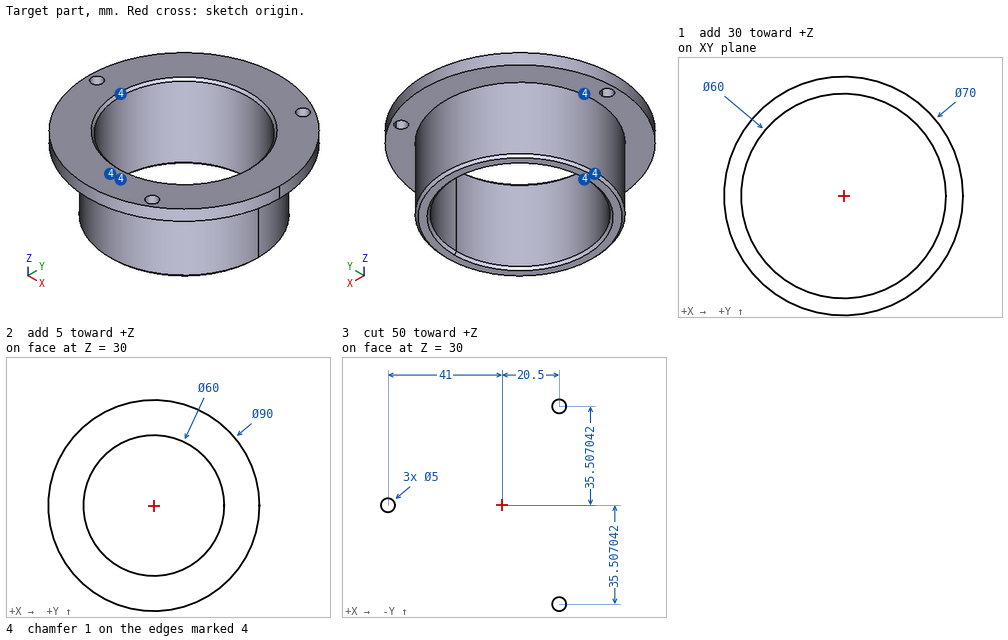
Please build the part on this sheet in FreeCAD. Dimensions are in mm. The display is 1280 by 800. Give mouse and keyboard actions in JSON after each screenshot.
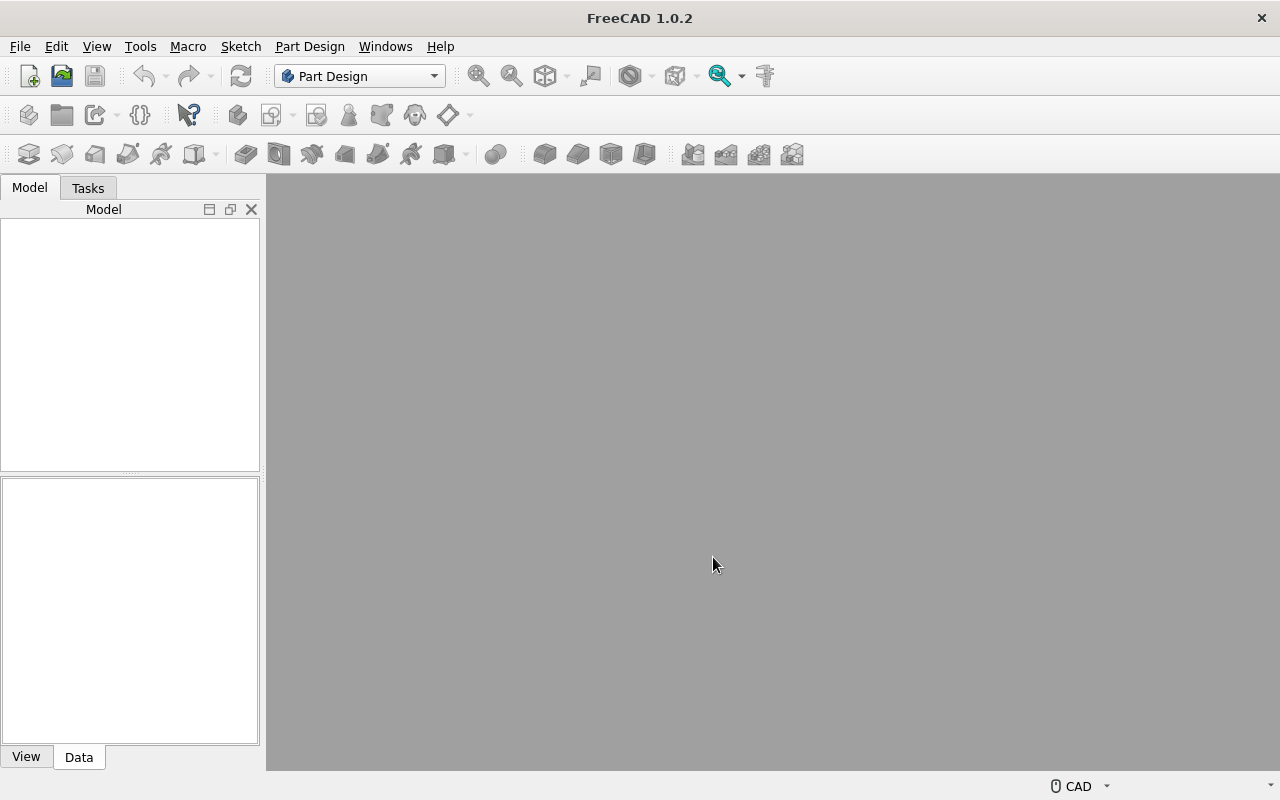
{"action": "key", "text": "ctrl+n"}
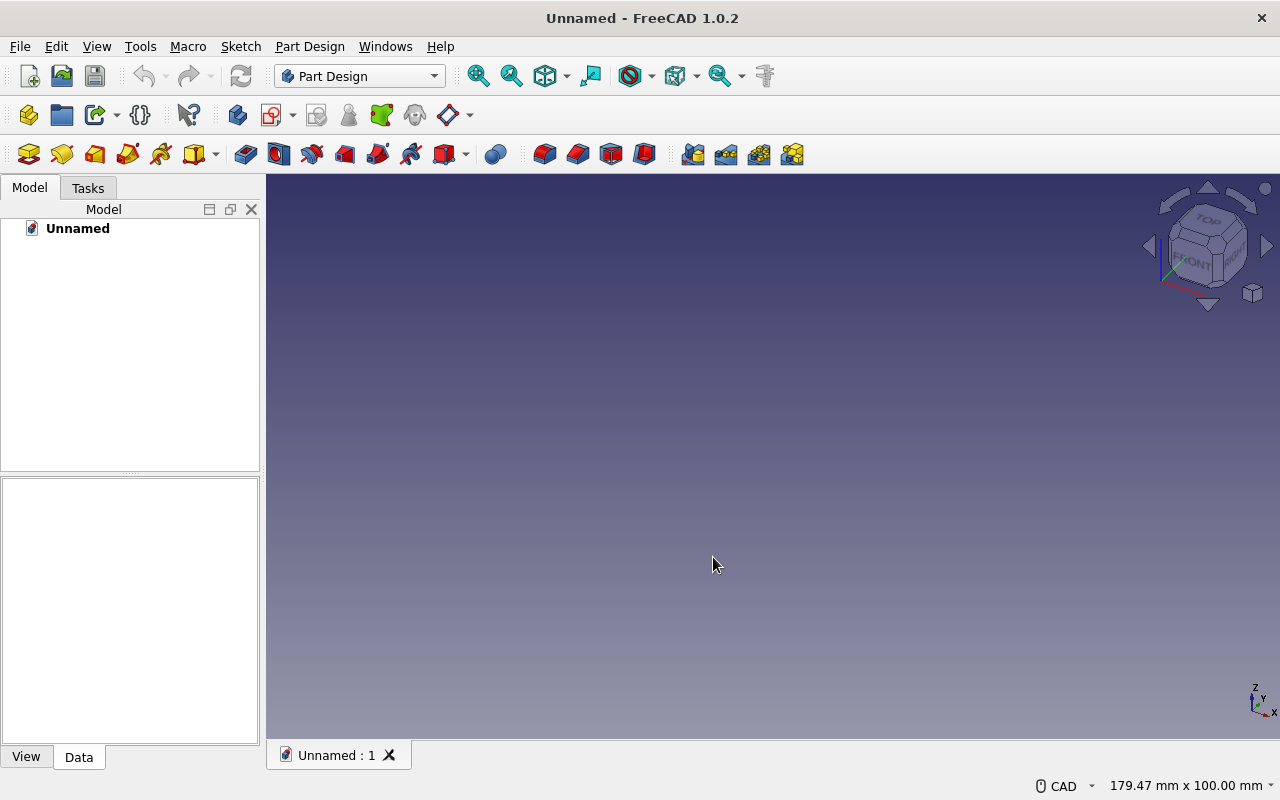
{"action": "left_click", "coordinate": [270, 116]}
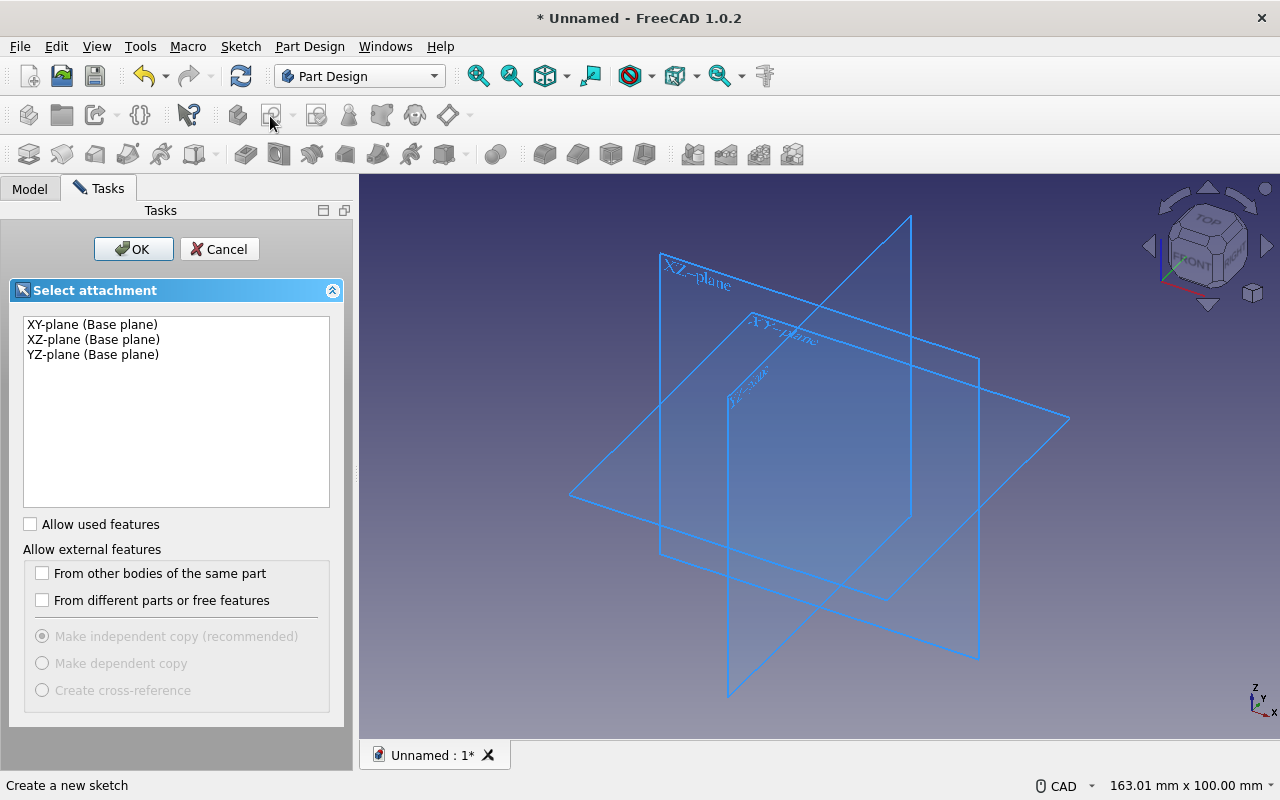
{"action": "left_click", "coordinate": [84, 324]}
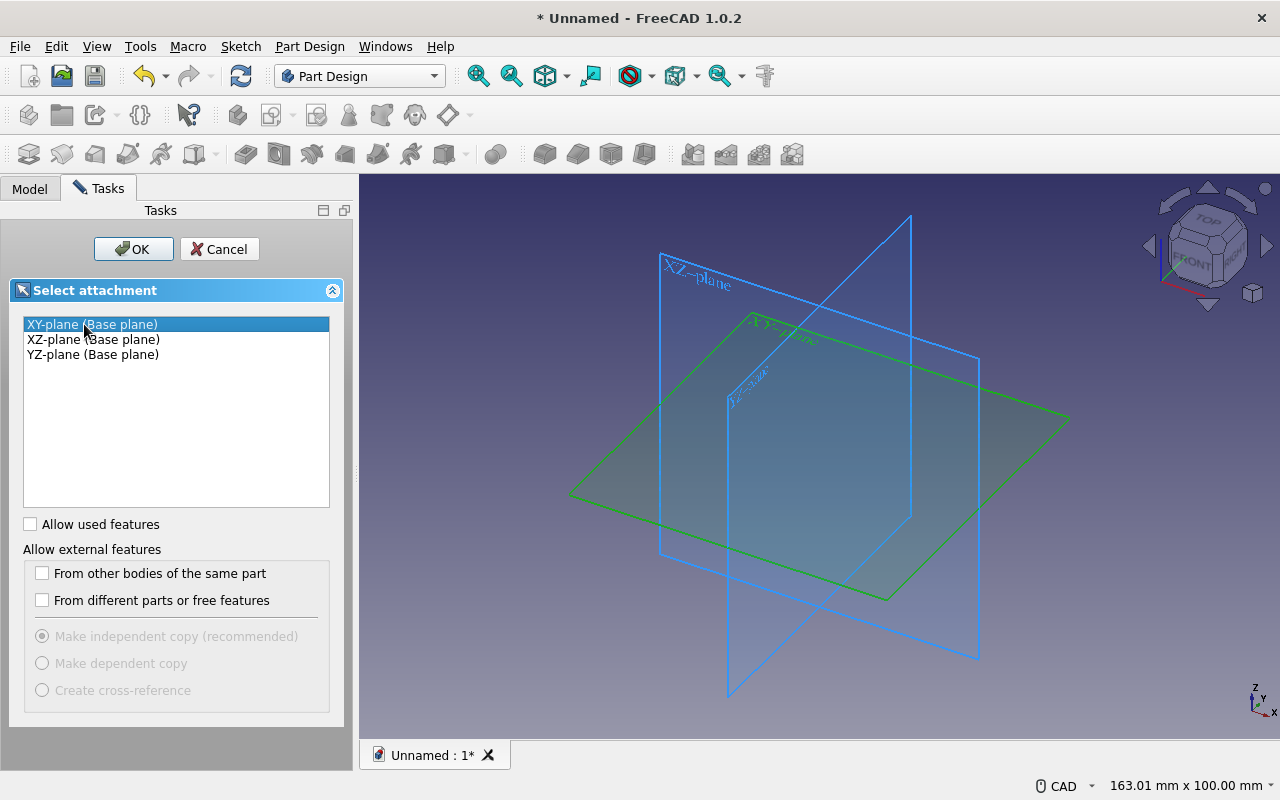
{"action": "left_click", "coordinate": [134, 249]}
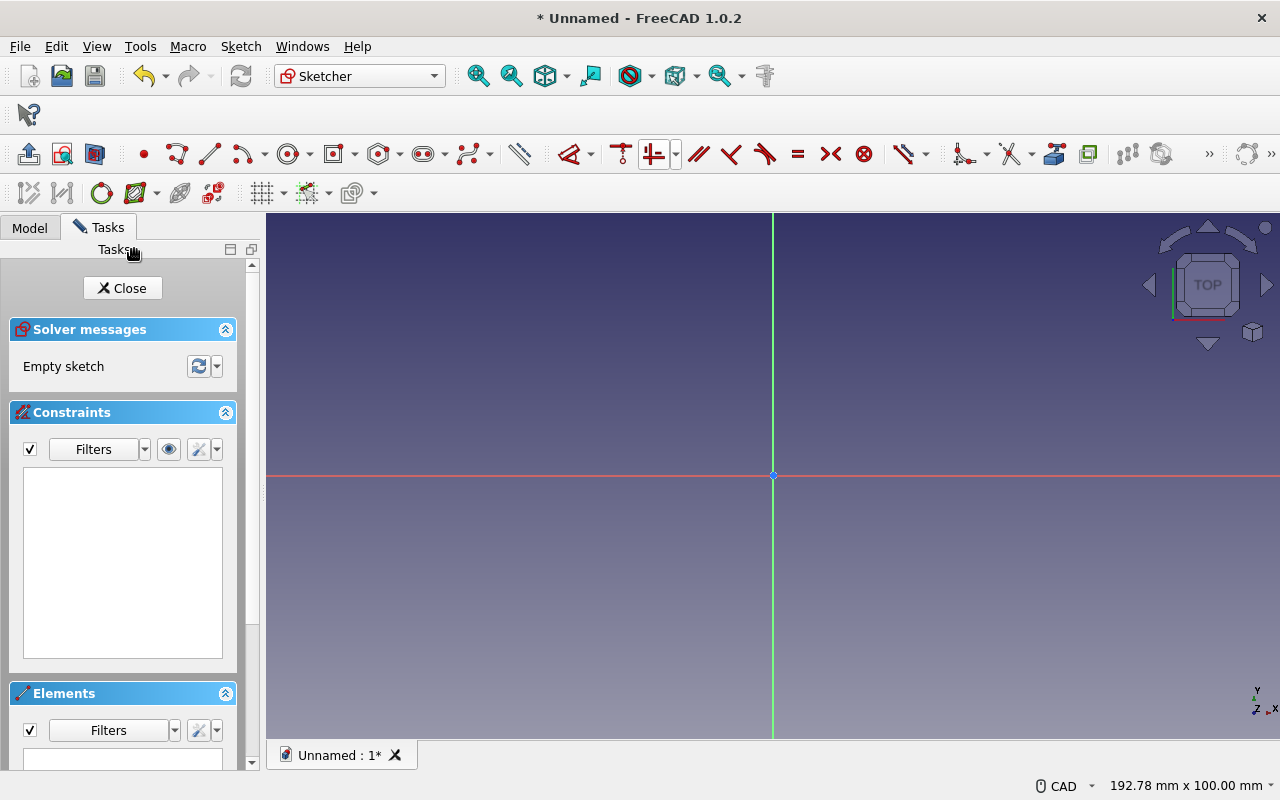
{"action": "left_click", "coordinate": [288, 154]}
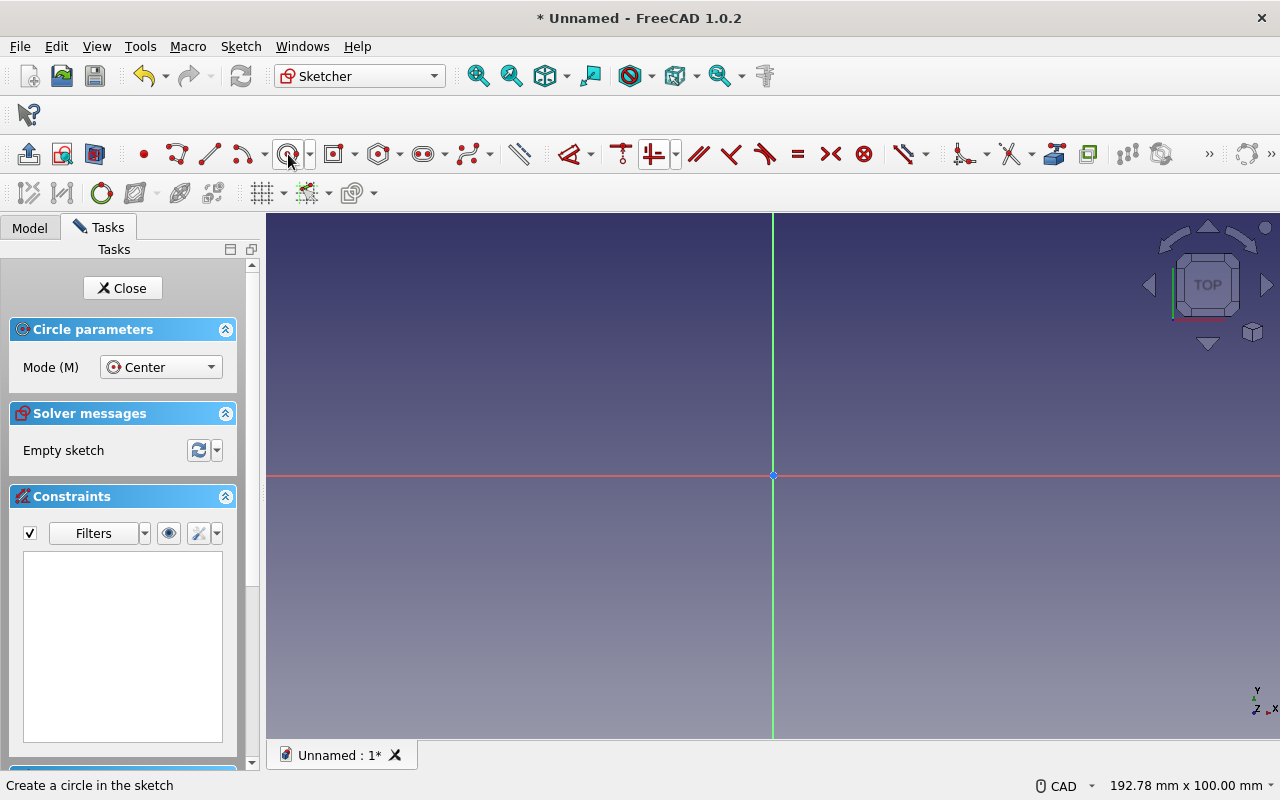
{"action": "left_click", "coordinate": [773, 476]}
{"action": "left_click", "coordinate": [903, 346]}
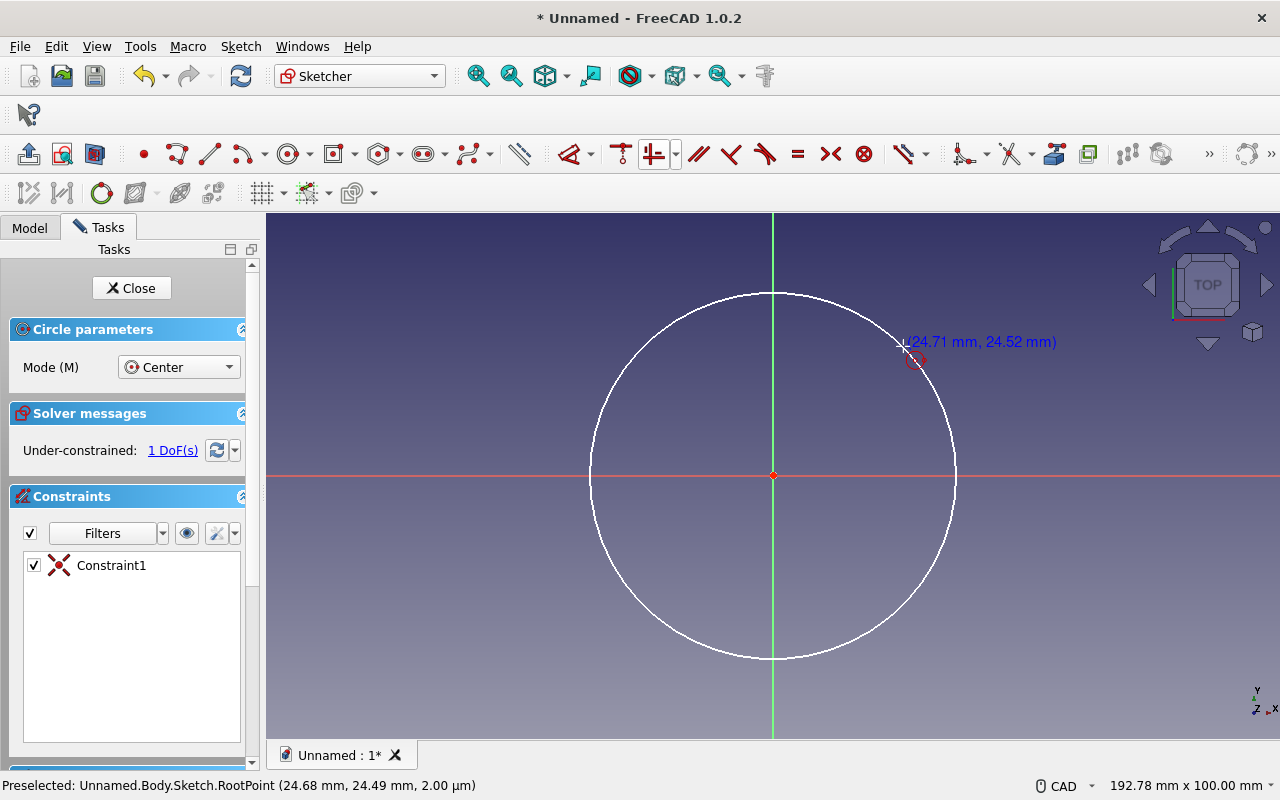
{"action": "left_click", "coordinate": [773, 476]}
{"action": "left_click", "coordinate": [885, 364]}
{"action": "key", "text": "Escape"}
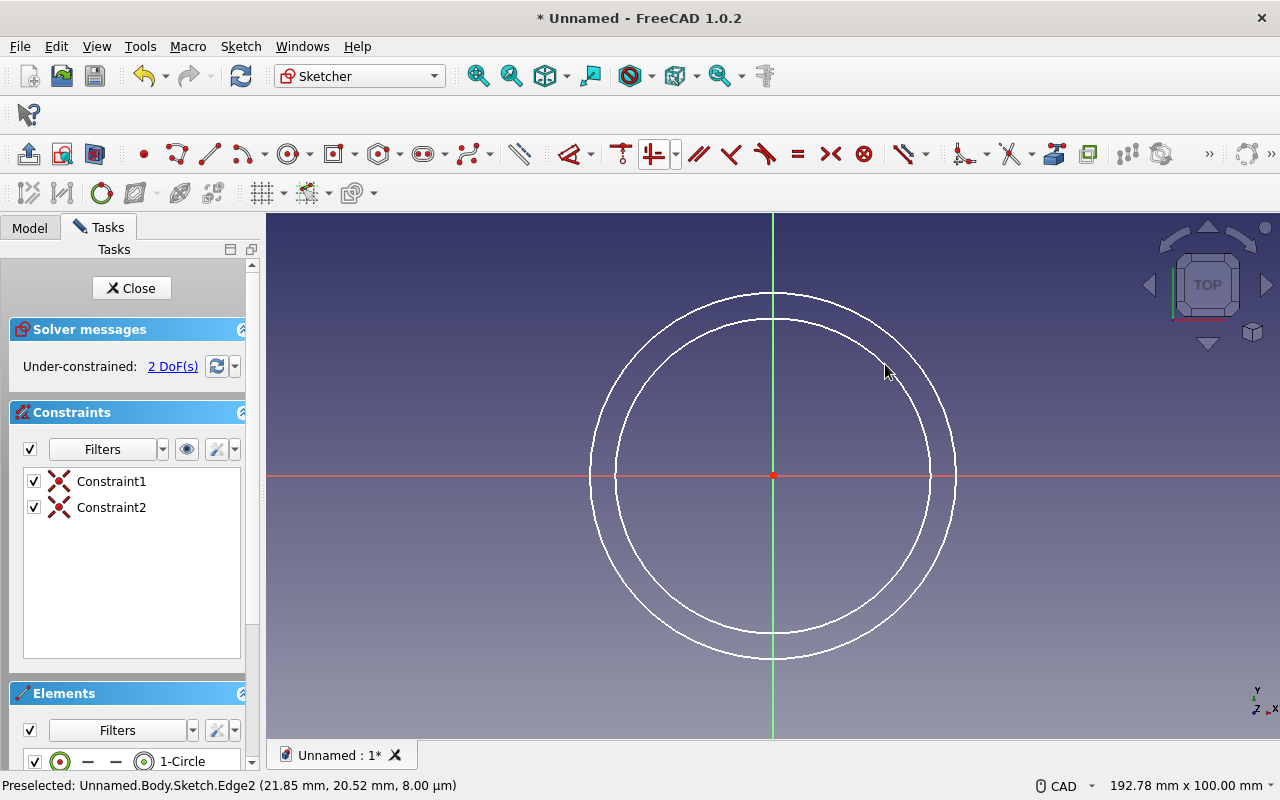
{"action": "left_click", "coordinate": [568, 154]}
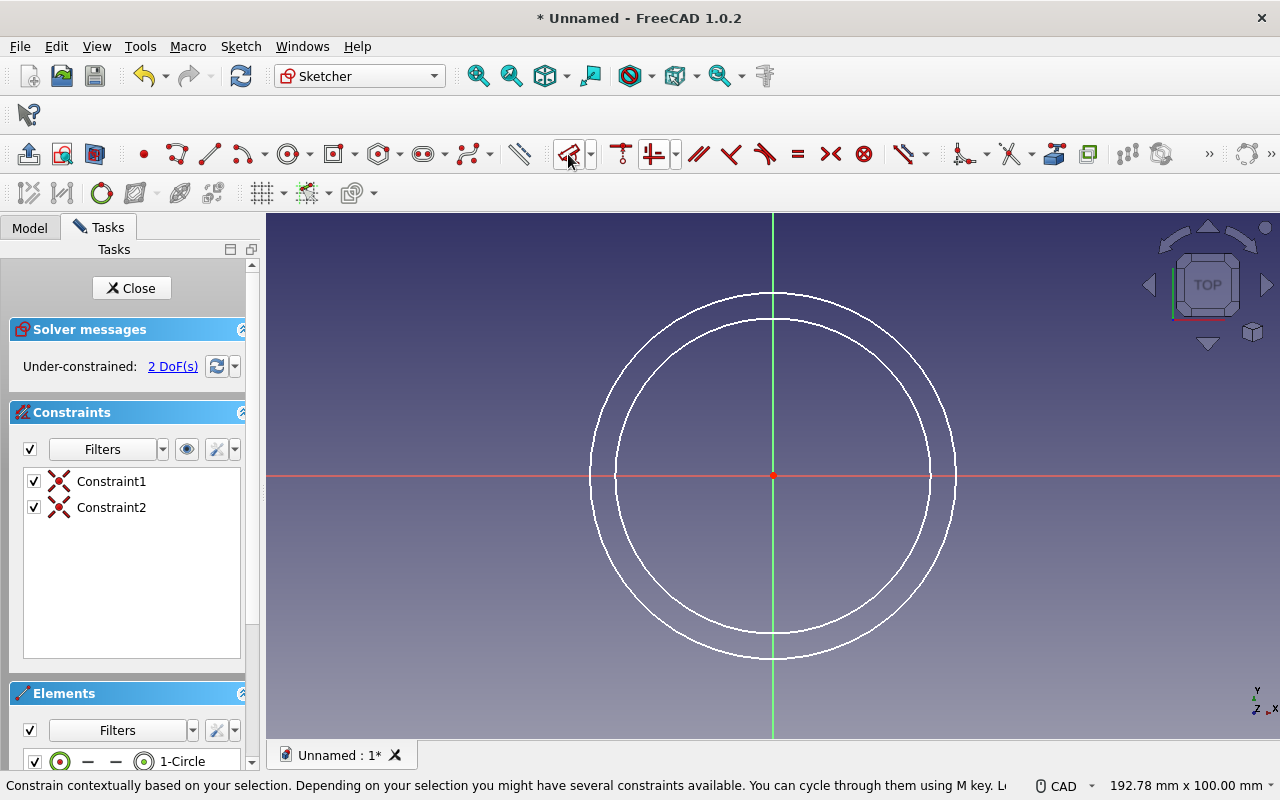
{"action": "left_click", "coordinate": [902, 346]}
{"action": "left_click", "coordinate": [925, 323]}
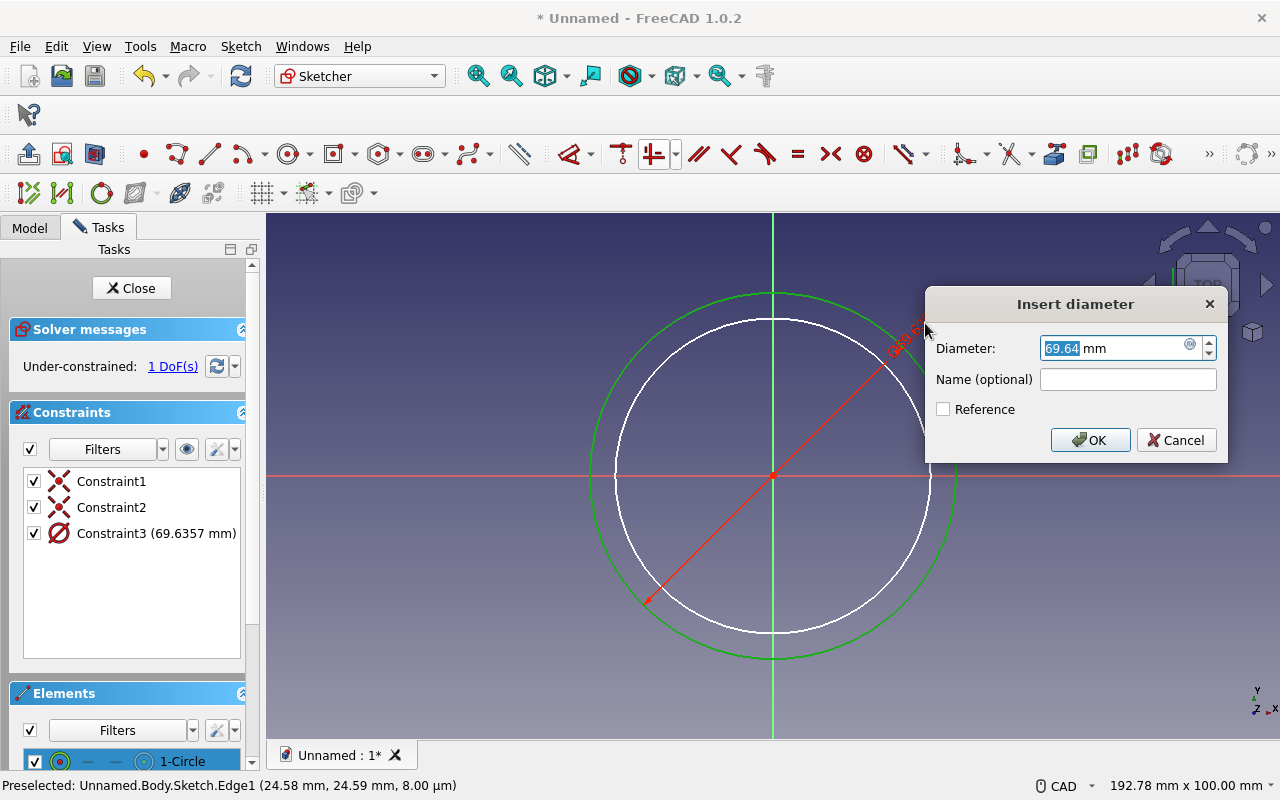
{"action": "type", "text": "70"}
{"action": "key", "text": "Return"}